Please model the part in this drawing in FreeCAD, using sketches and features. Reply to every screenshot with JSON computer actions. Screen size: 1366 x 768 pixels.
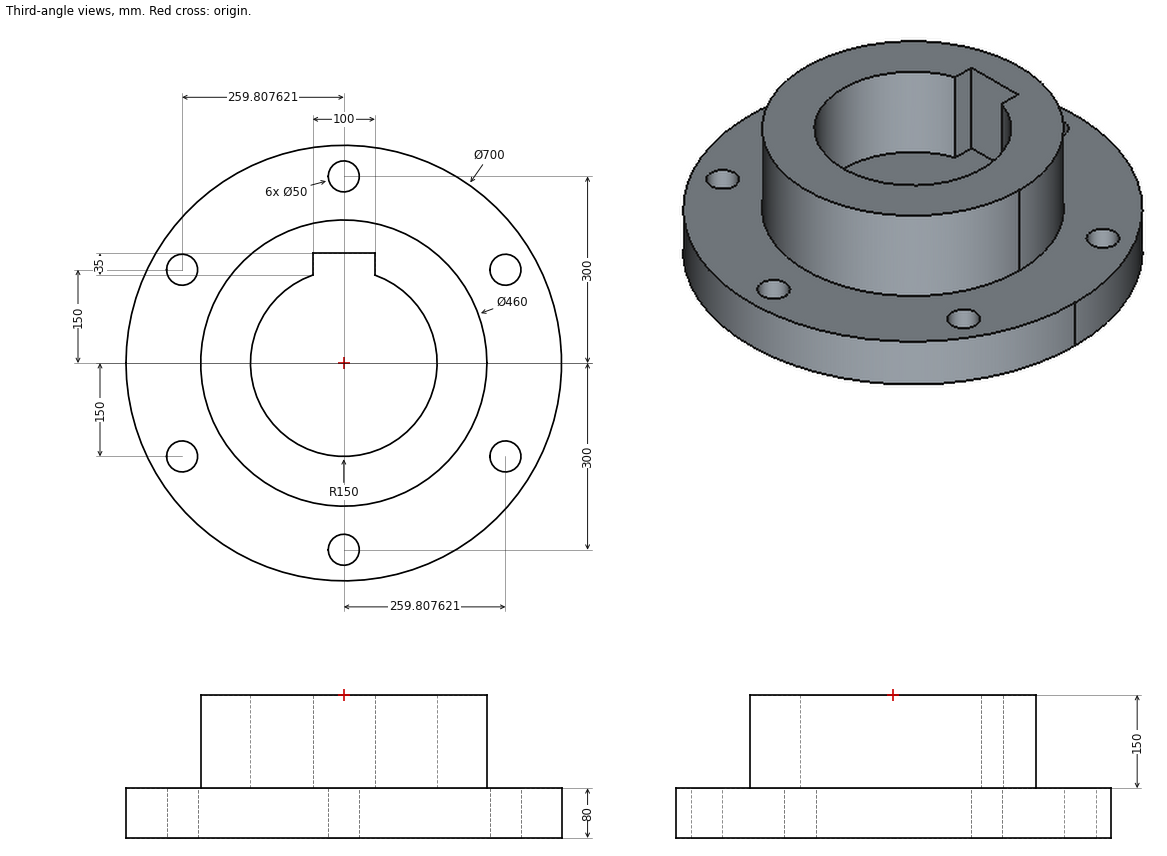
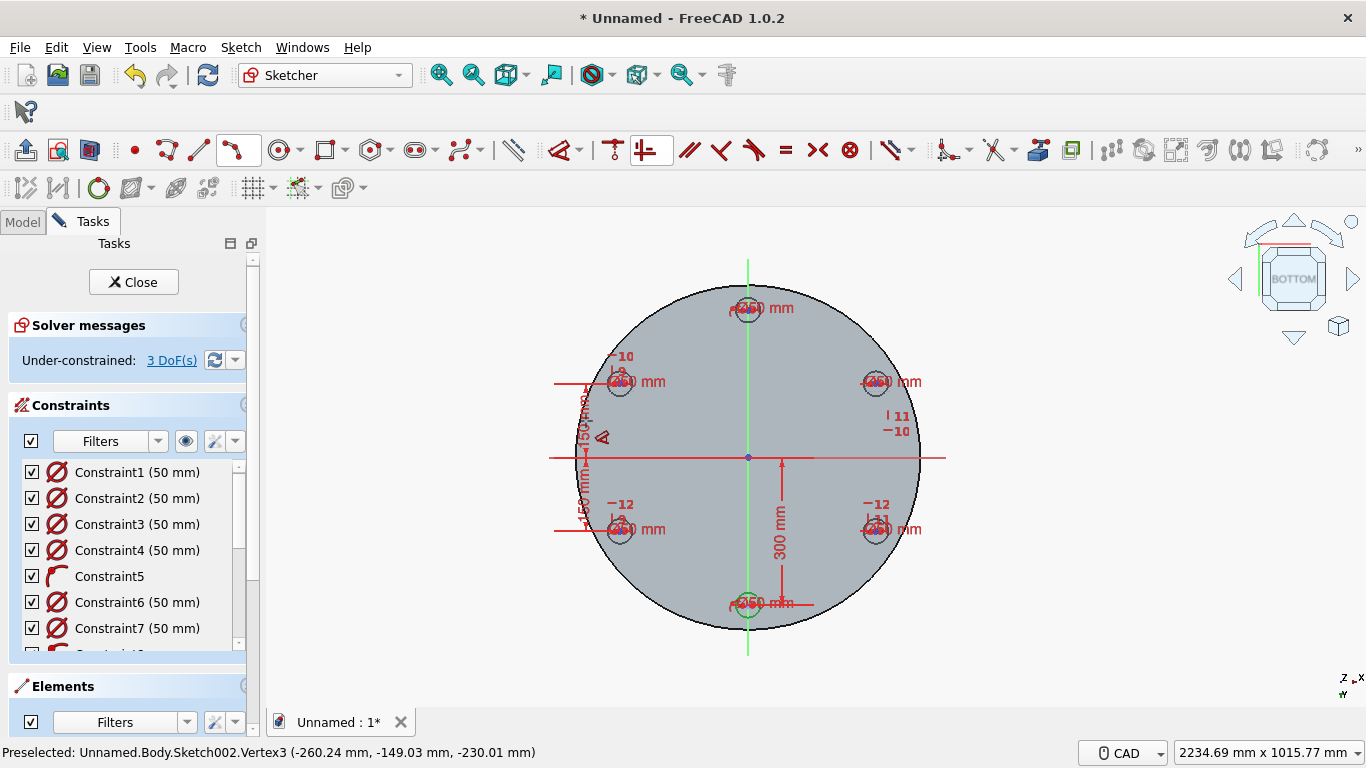
{"action": "left_click", "coordinate": [748, 310]}
{"action": "left_click", "coordinate": [782, 384]}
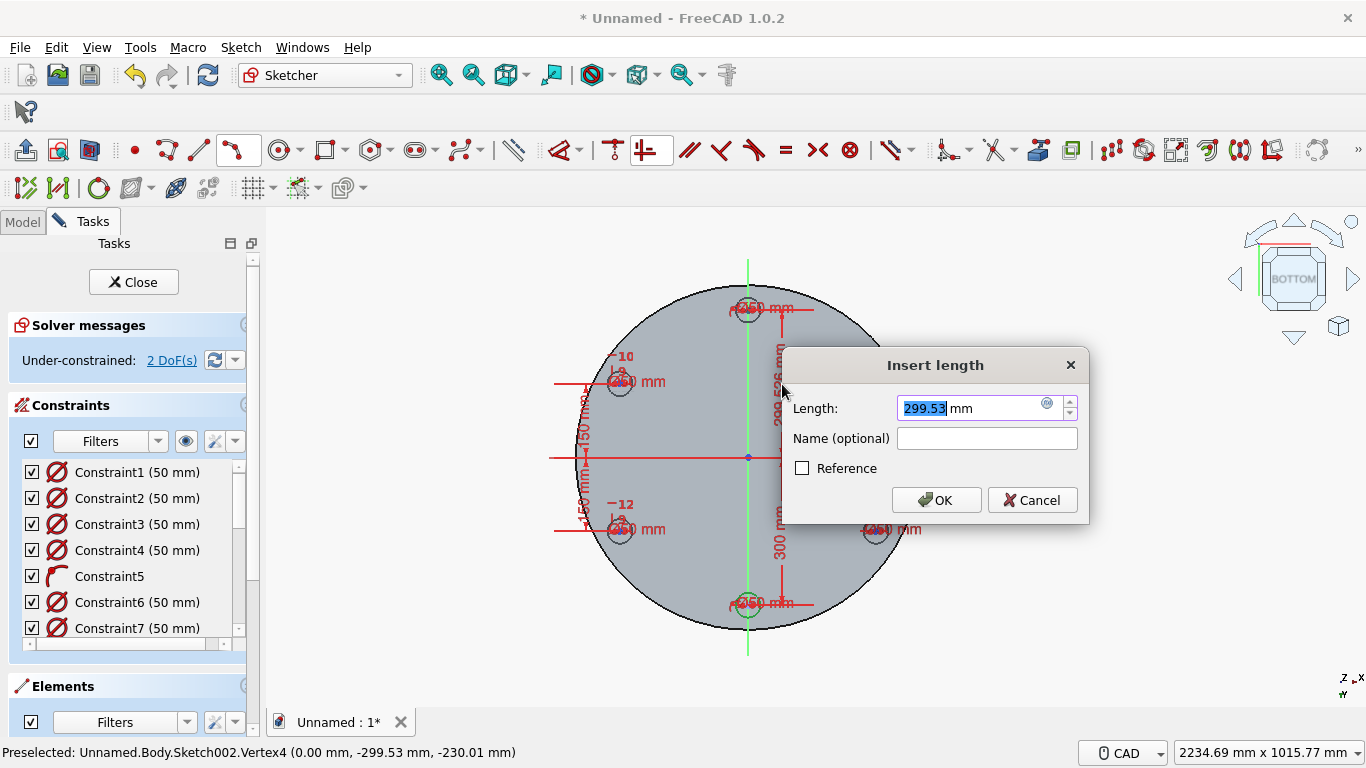
{"action": "type", "text": "300"}
{"action": "key", "text": "Return"}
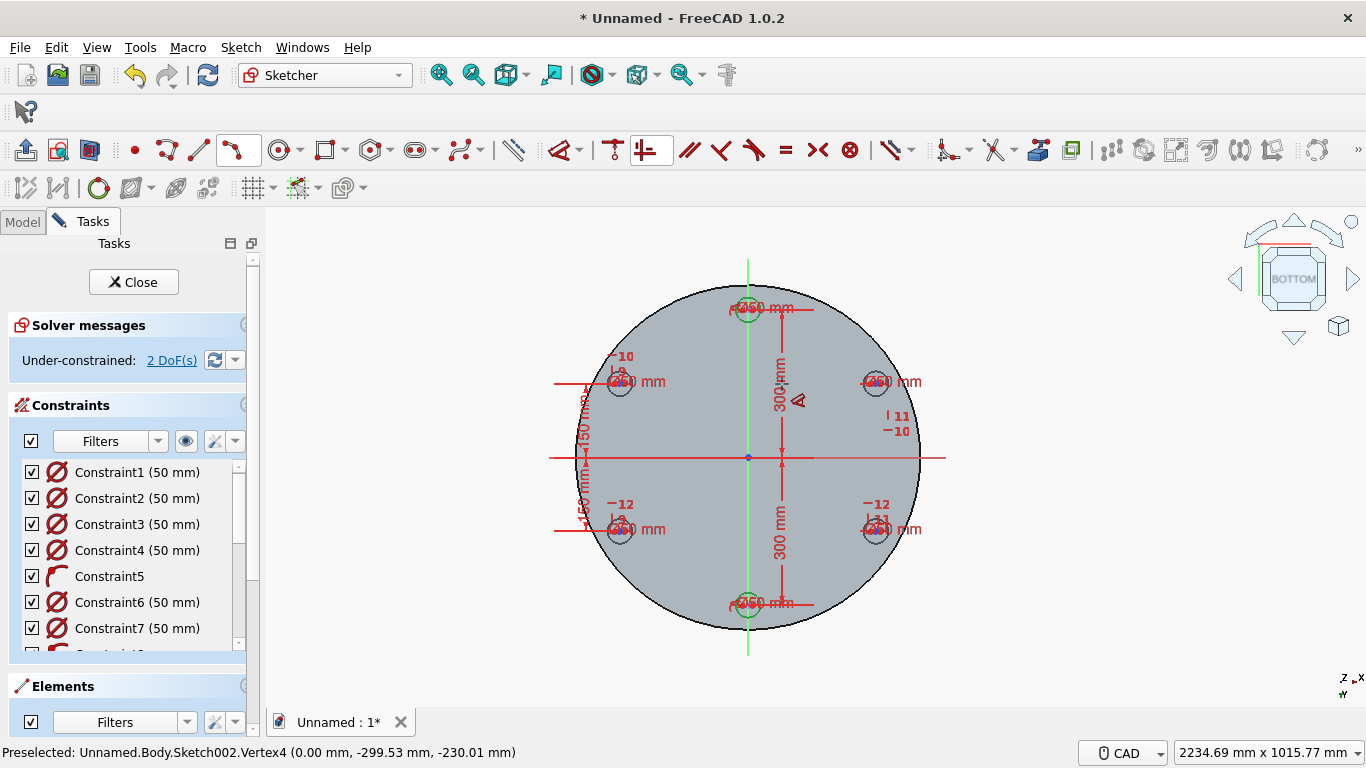
{"action": "left_click", "coordinate": [620, 531]}
{"action": "left_click", "coordinate": [684, 565]}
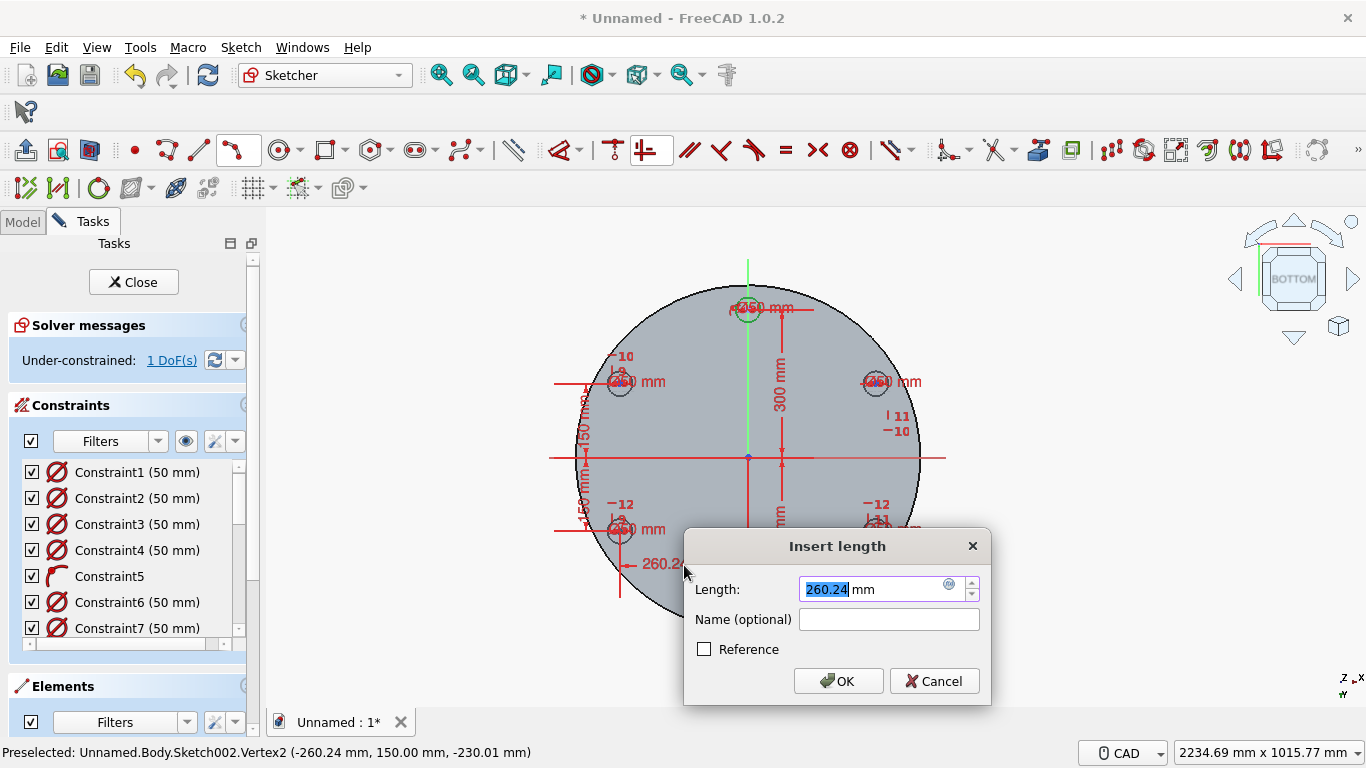
{"action": "type", "text": "259.807621"}
{"action": "key", "text": "Return"}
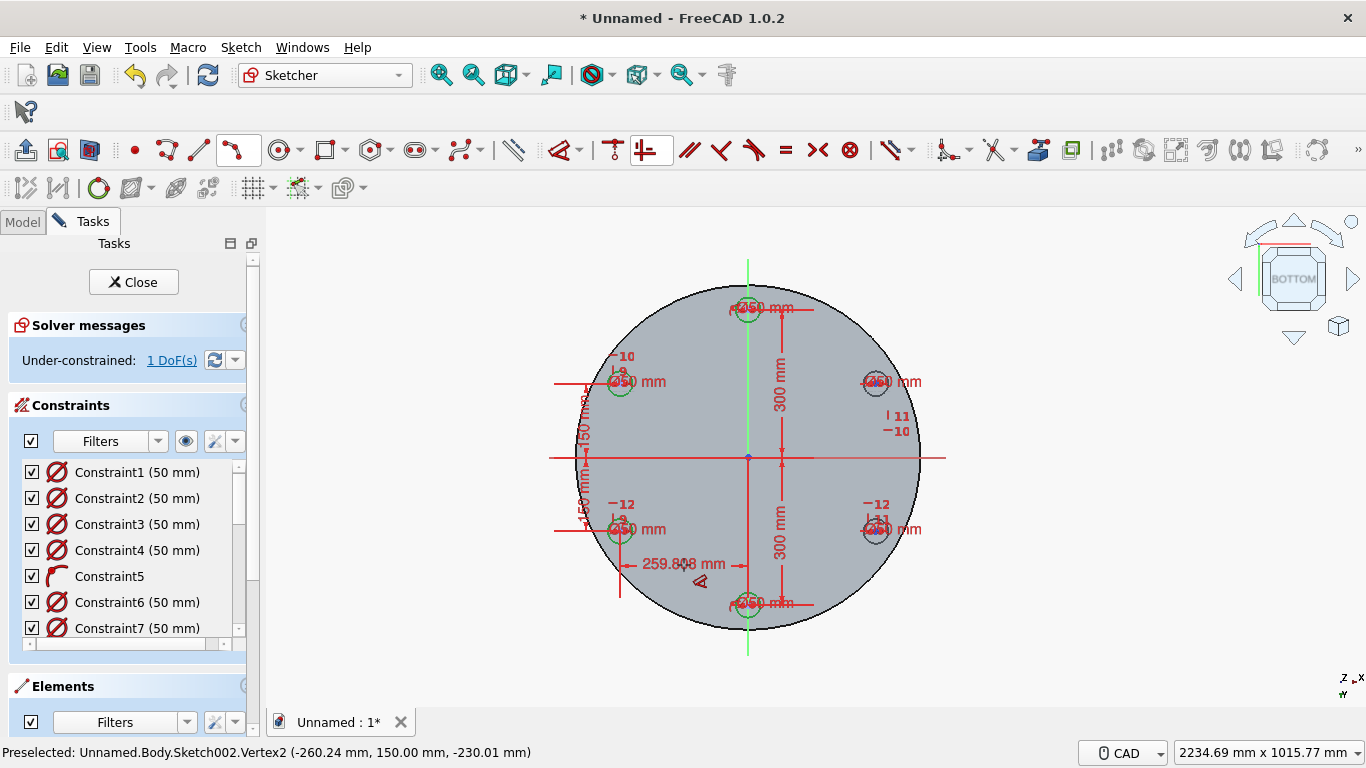
{"action": "left_click", "coordinate": [876, 384]}
{"action": "left_click", "coordinate": [812, 350]}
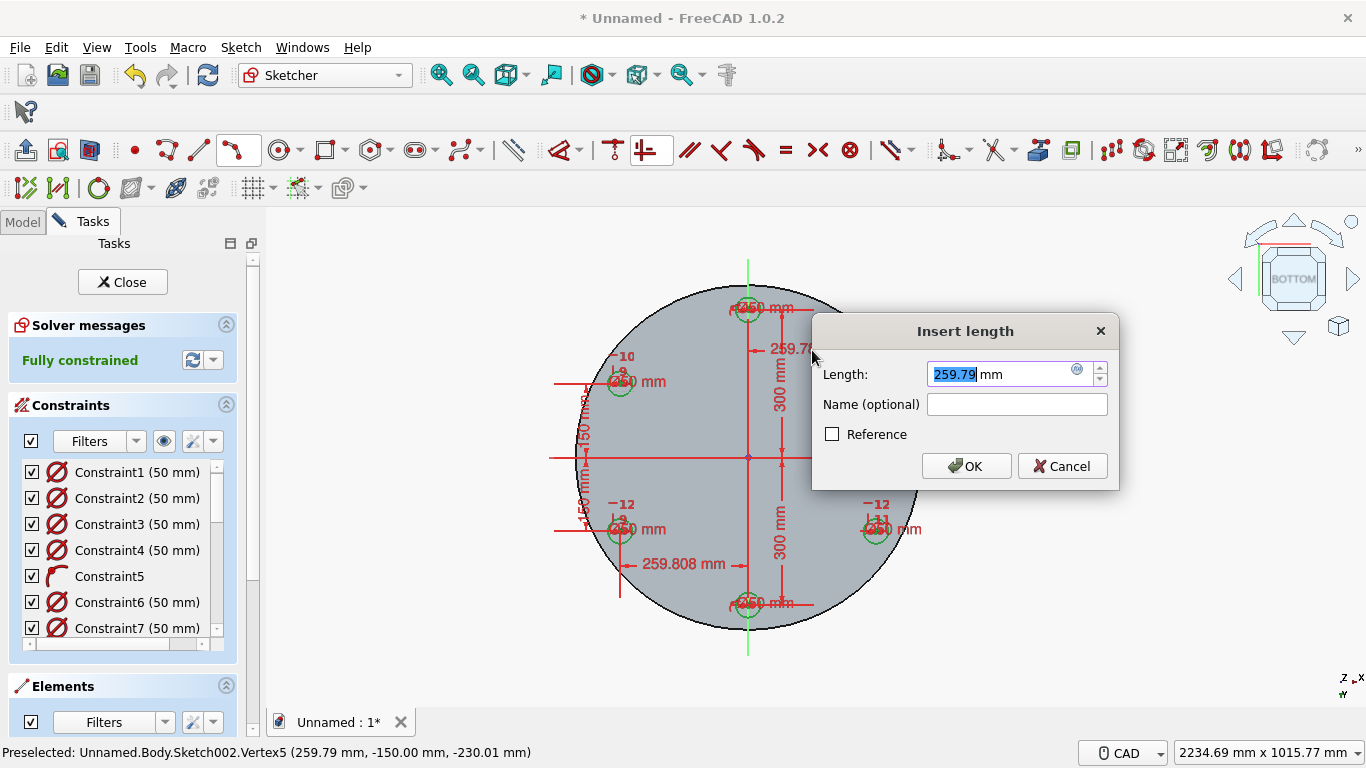
{"action": "type", "text": "259.807621"}
{"action": "key", "text": "Return"}
{"action": "key", "text": "Escape"}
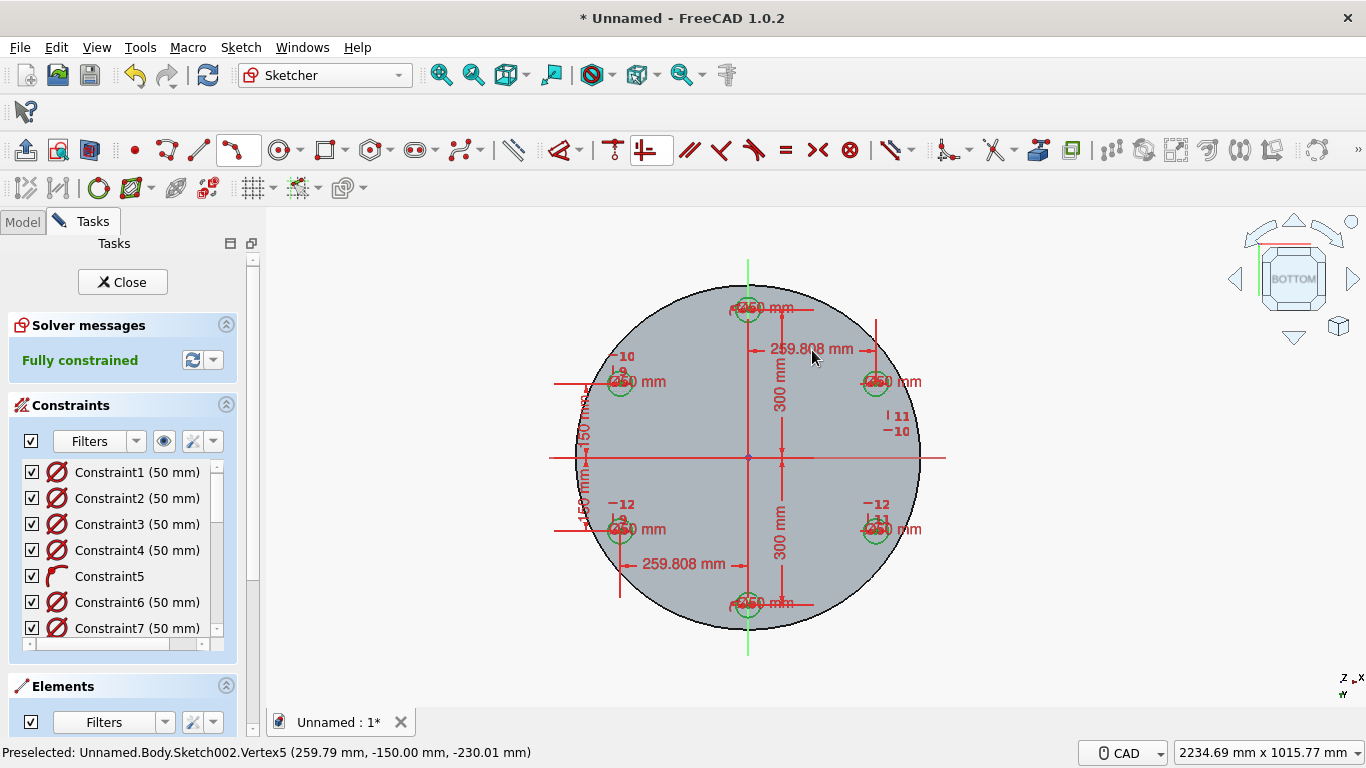
{"action": "left_click", "coordinate": [123, 282]}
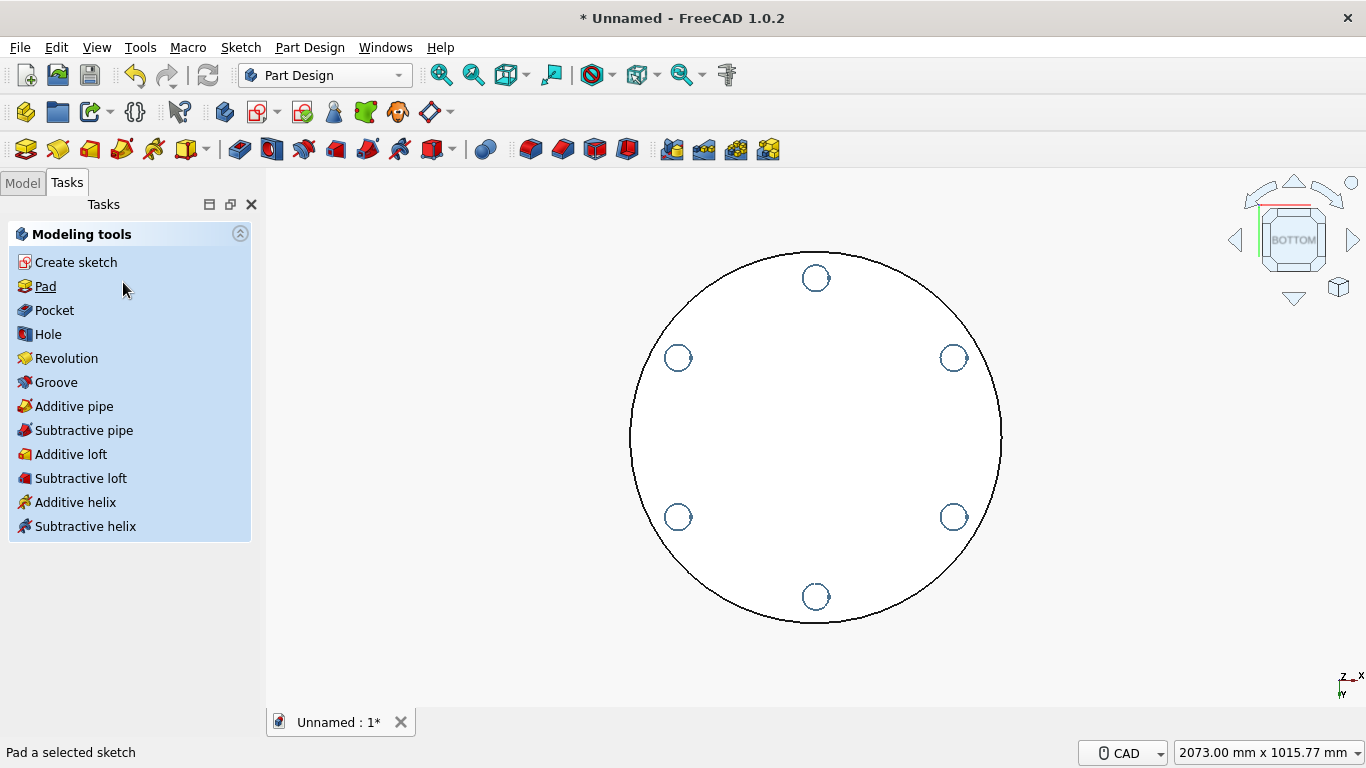
{"action": "left_click", "coordinate": [240, 150]}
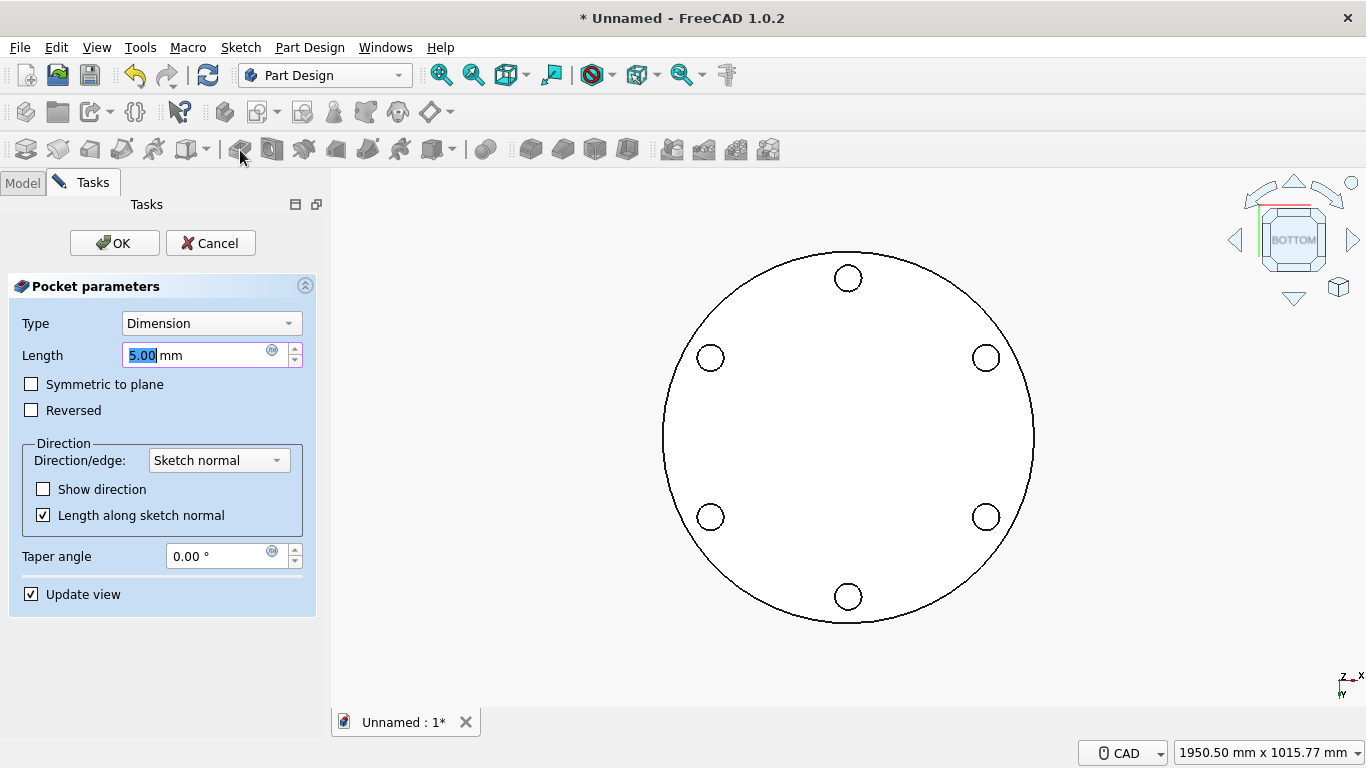
{"action": "left_click", "coordinate": [212, 324]}